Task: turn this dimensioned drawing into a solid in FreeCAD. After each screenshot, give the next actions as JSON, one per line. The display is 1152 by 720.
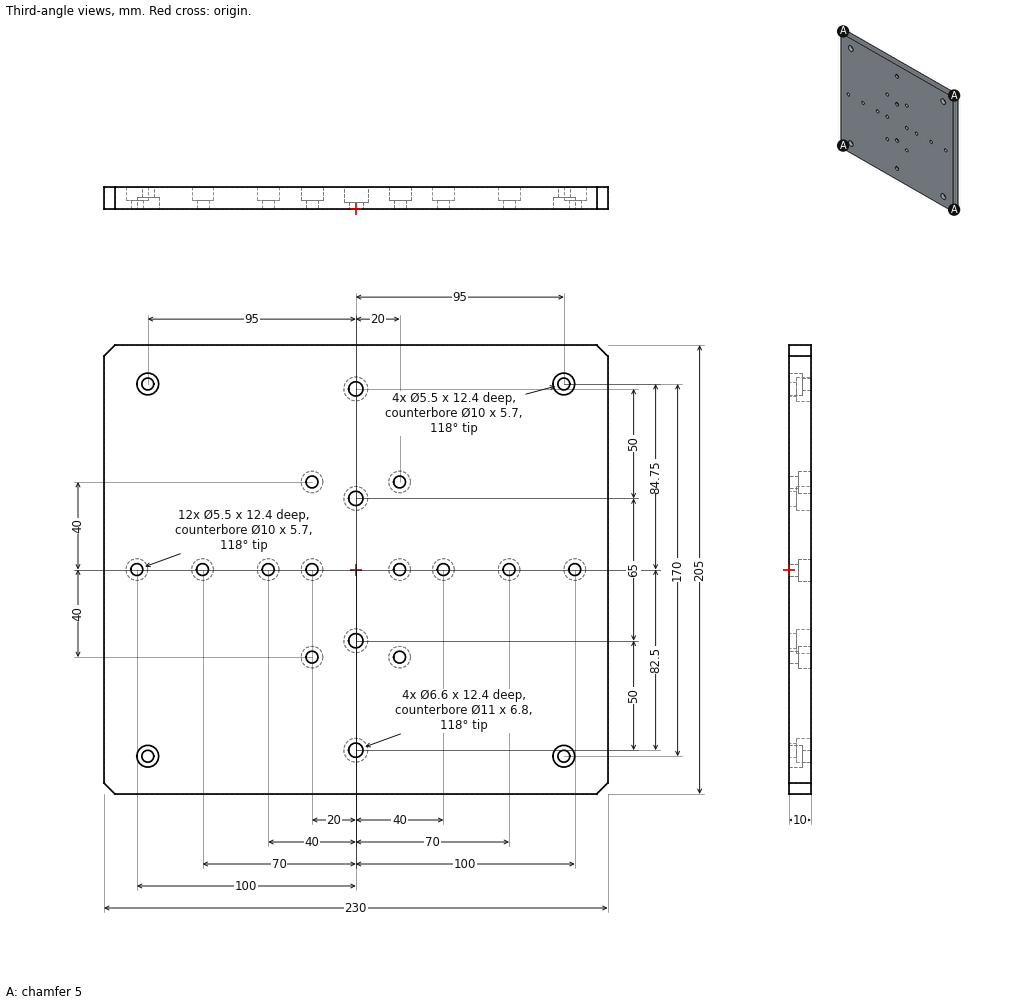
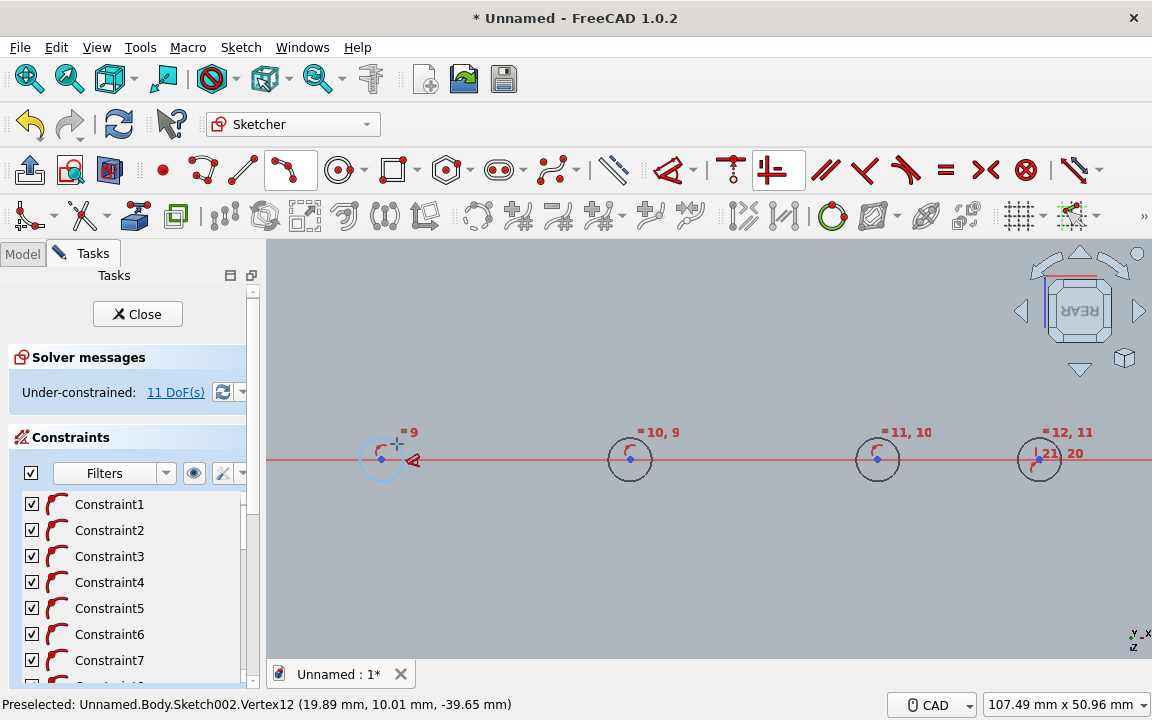
{"action": "left_click", "coordinate": [397, 444]}
{"action": "left_click", "coordinate": [419, 421]}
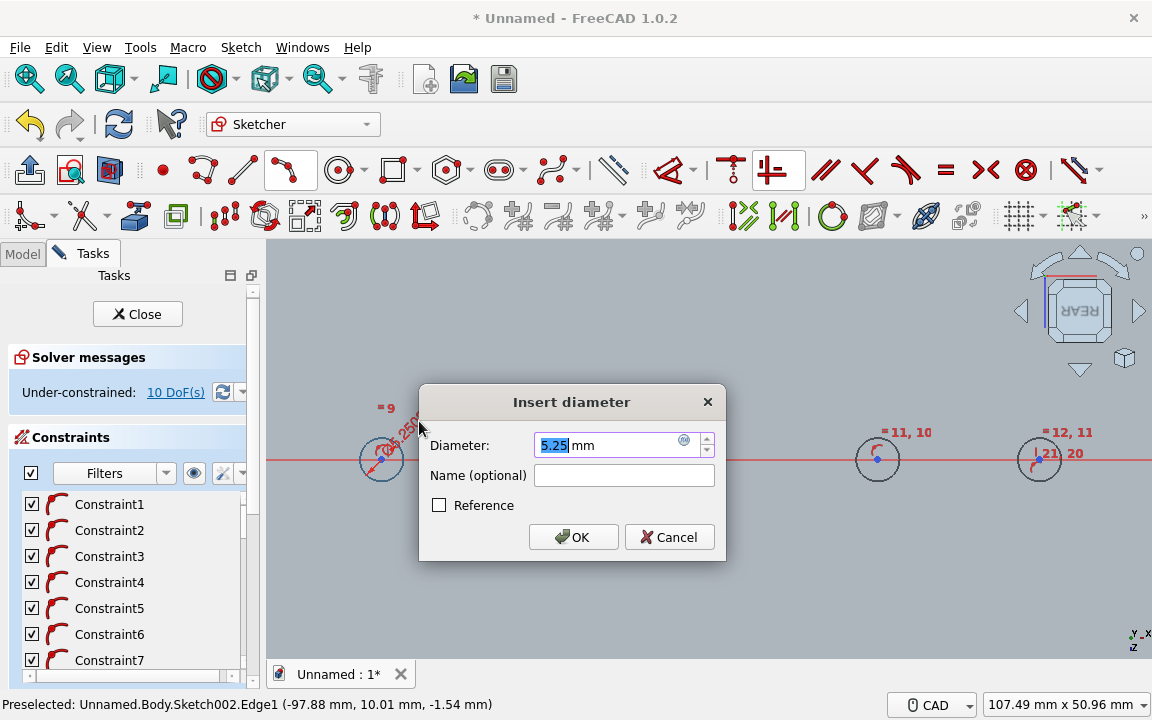
{"action": "type", "text": "5.5"}
{"action": "key", "text": "Return"}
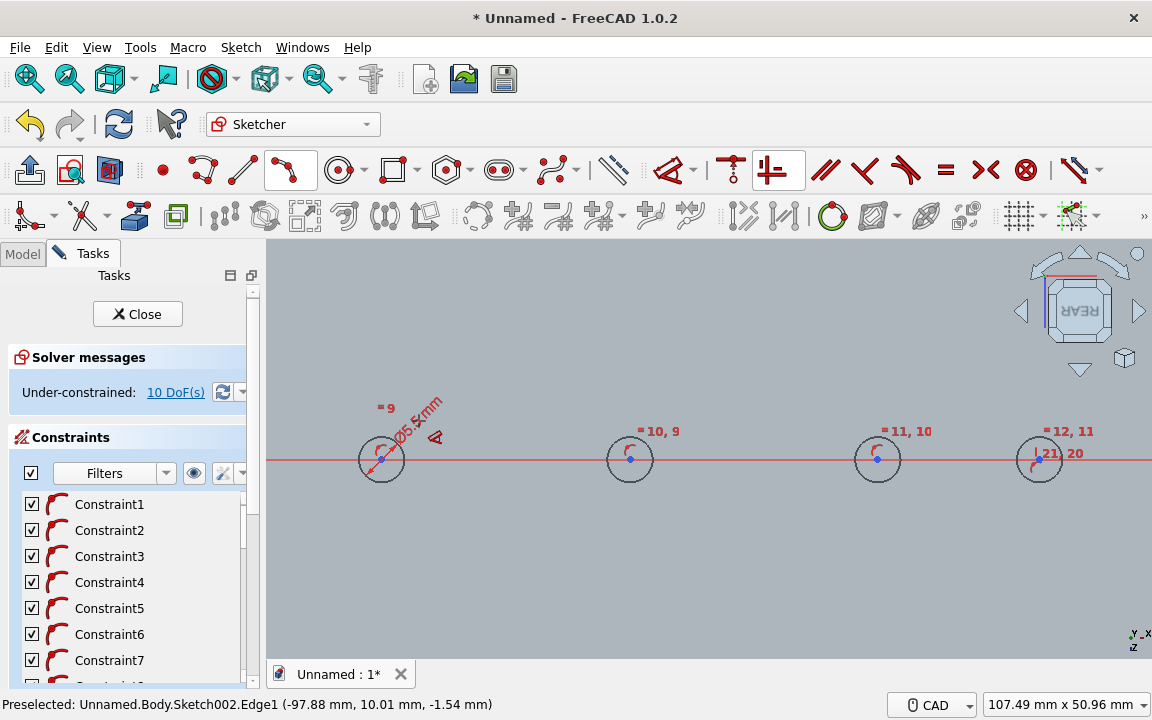
{"action": "left_click", "coordinate": [630, 460]}
{"action": "left_click", "coordinate": [809, 494]}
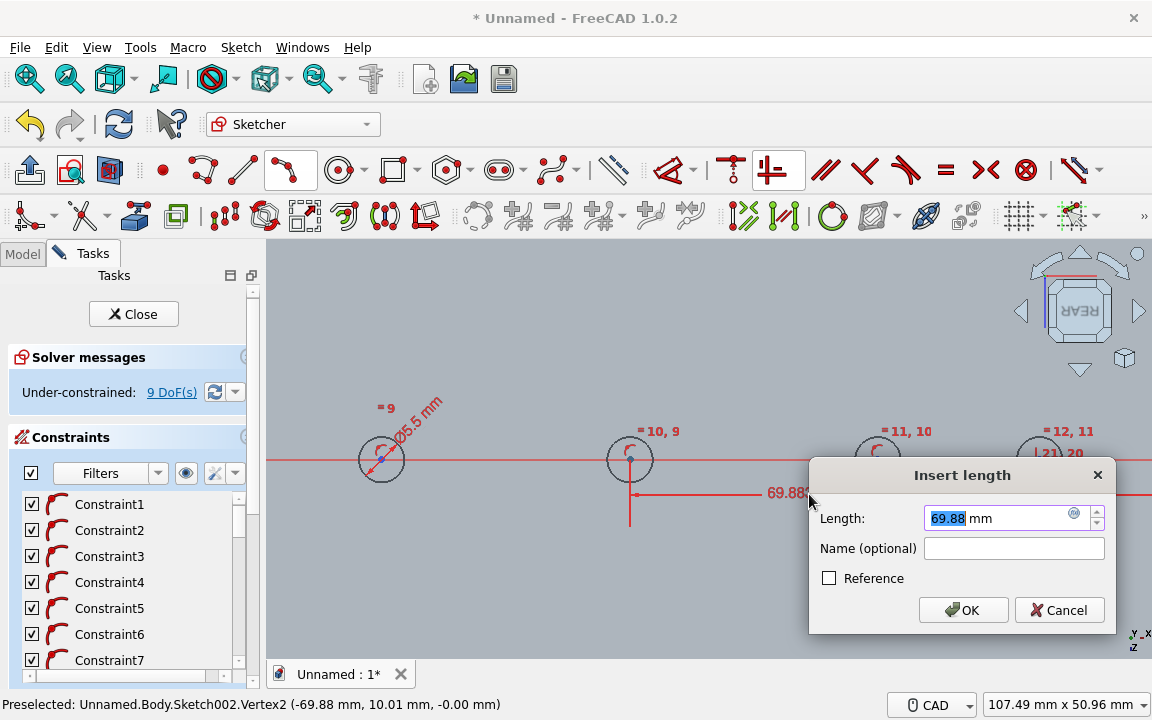
{"action": "type", "text": "70"}
{"action": "key", "text": "Return"}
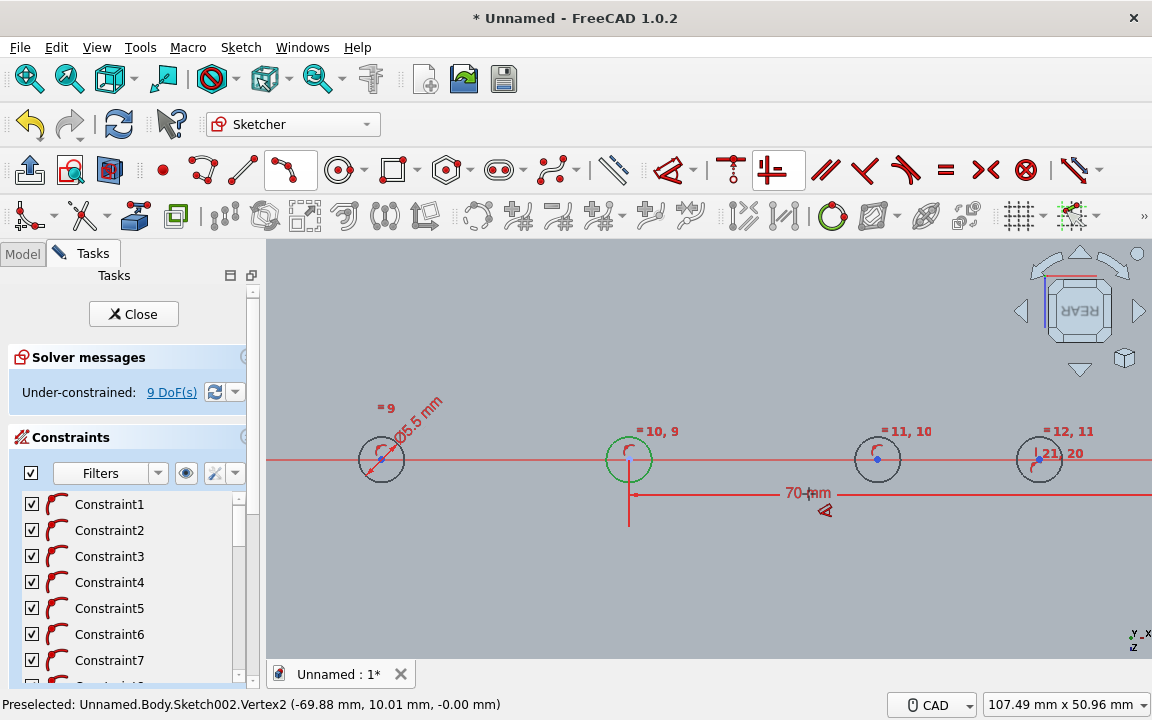
{"action": "left_click", "coordinate": [878, 460]}
{"action": "left_click", "coordinate": [932, 494]}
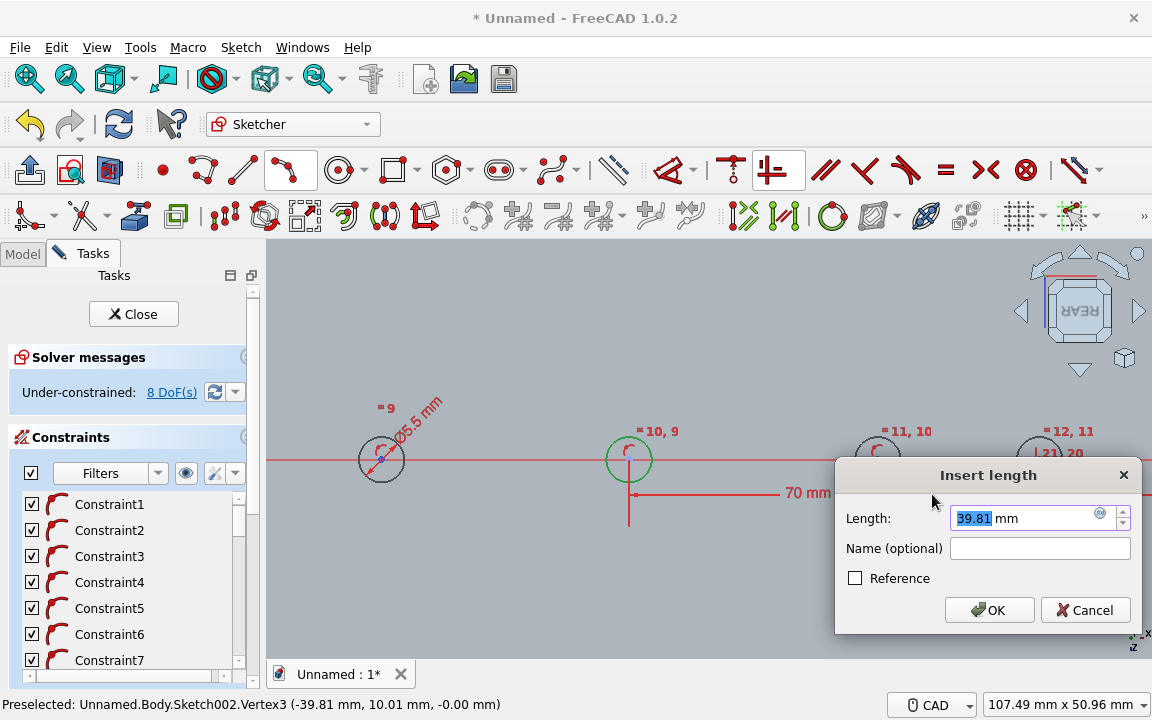
{"action": "type", "text": "40"}
{"action": "key", "text": "Return"}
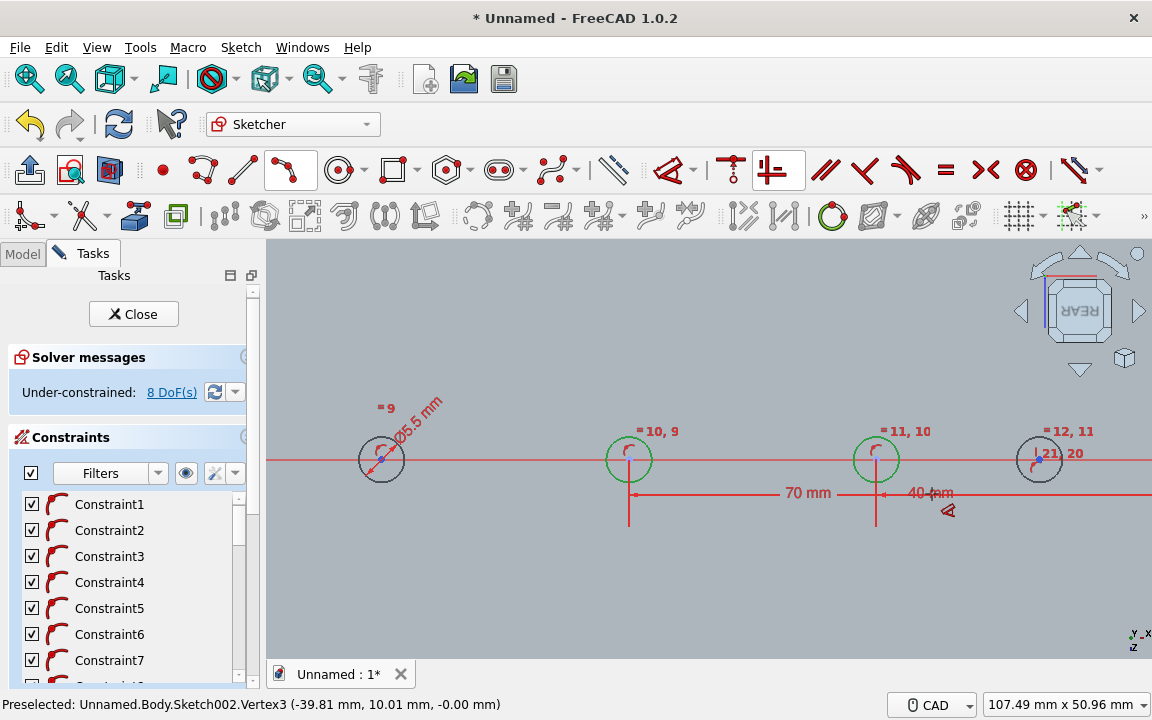
{"action": "scroll", "coordinate": [397, 444], "scroll_direction": "down", "scroll_amount": 6}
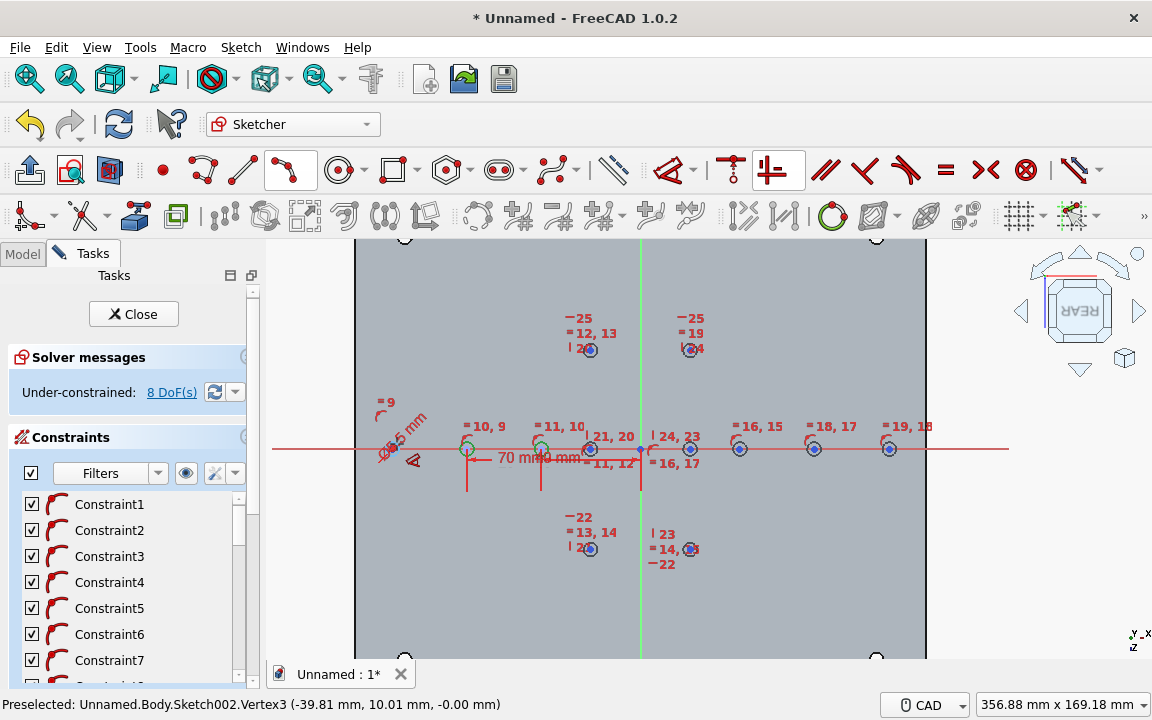
{"action": "left_click", "coordinate": [591, 449]}
{"action": "left_click", "coordinate": [616, 483]}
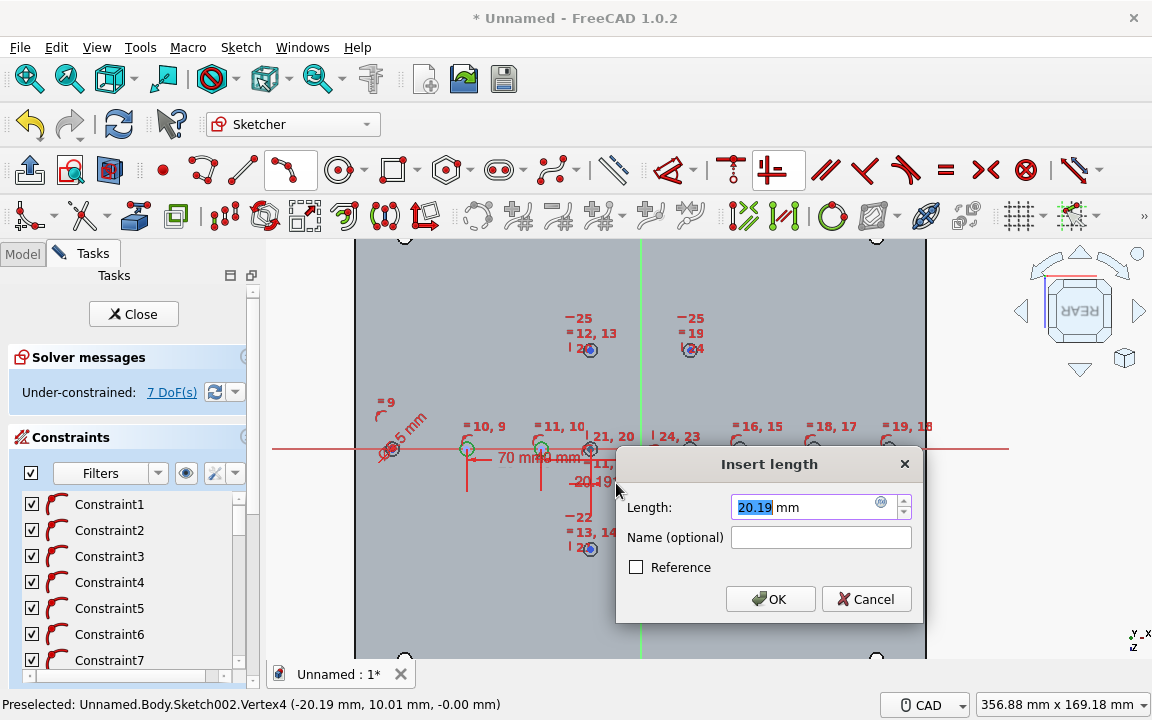
{"action": "type", "text": "20"}
{"action": "key", "text": "Return"}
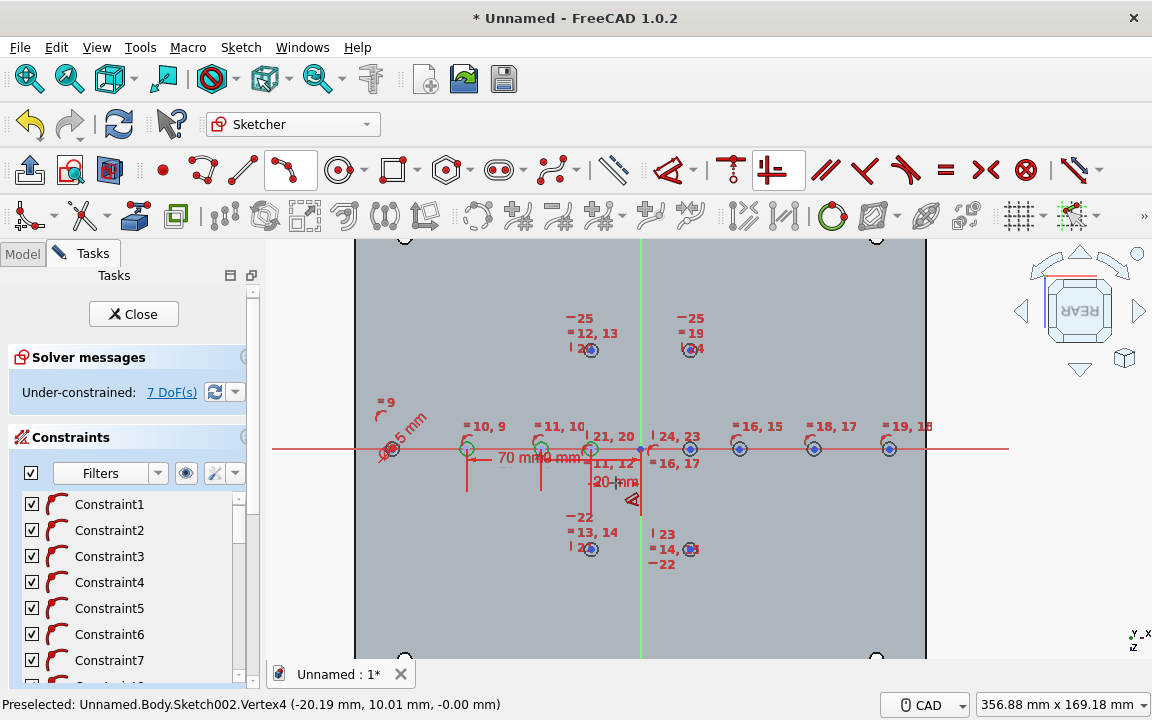
{"action": "left_click", "coordinate": [591, 351]}
{"action": "left_click", "coordinate": [557, 400]}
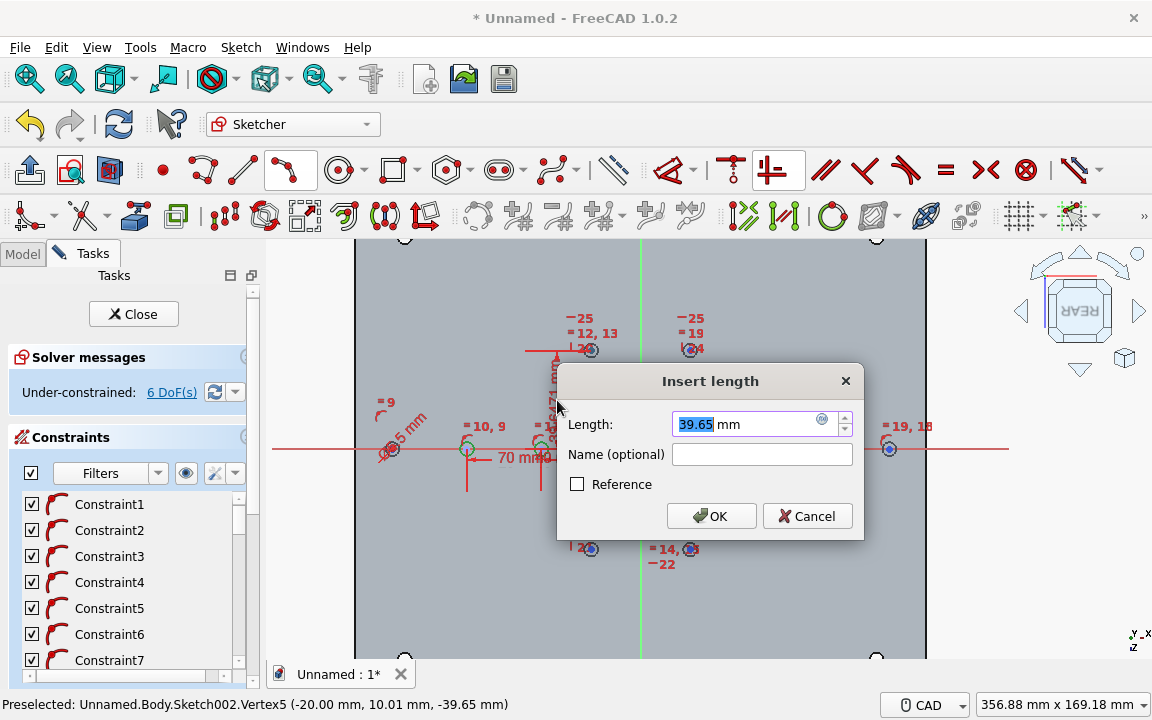
{"action": "type", "text": "40"}
{"action": "key", "text": "Return"}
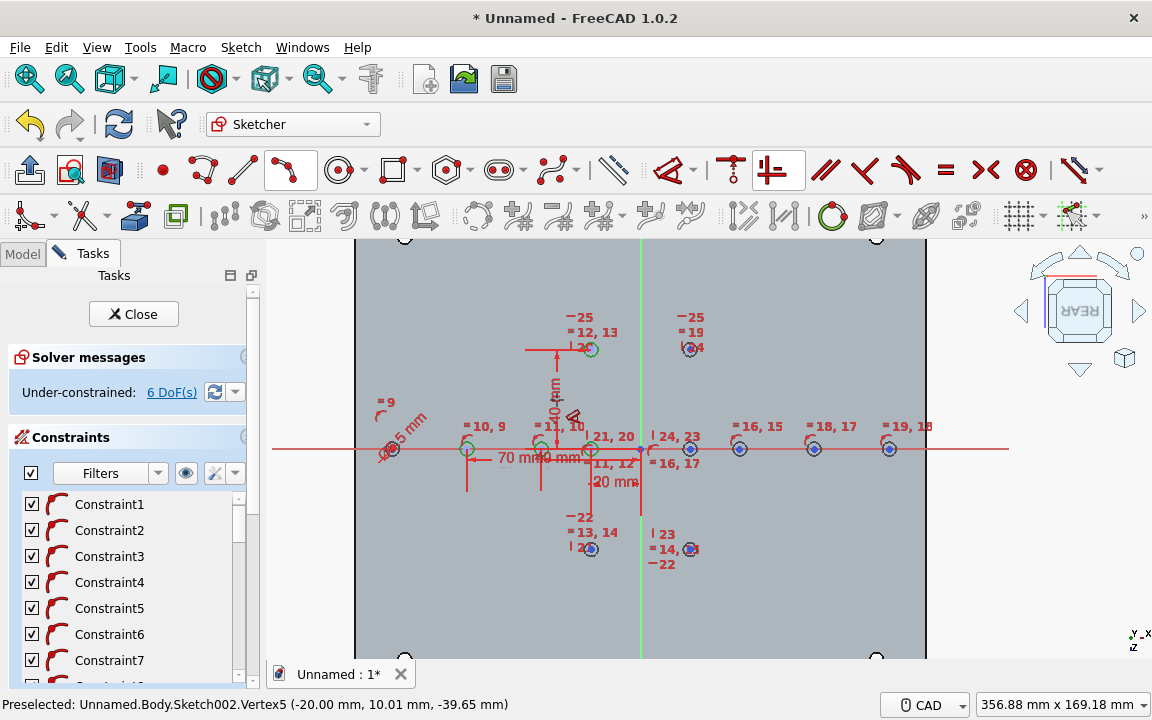
{"action": "left_click", "coordinate": [591, 550]}
{"action": "left_click", "coordinate": [557, 523]}